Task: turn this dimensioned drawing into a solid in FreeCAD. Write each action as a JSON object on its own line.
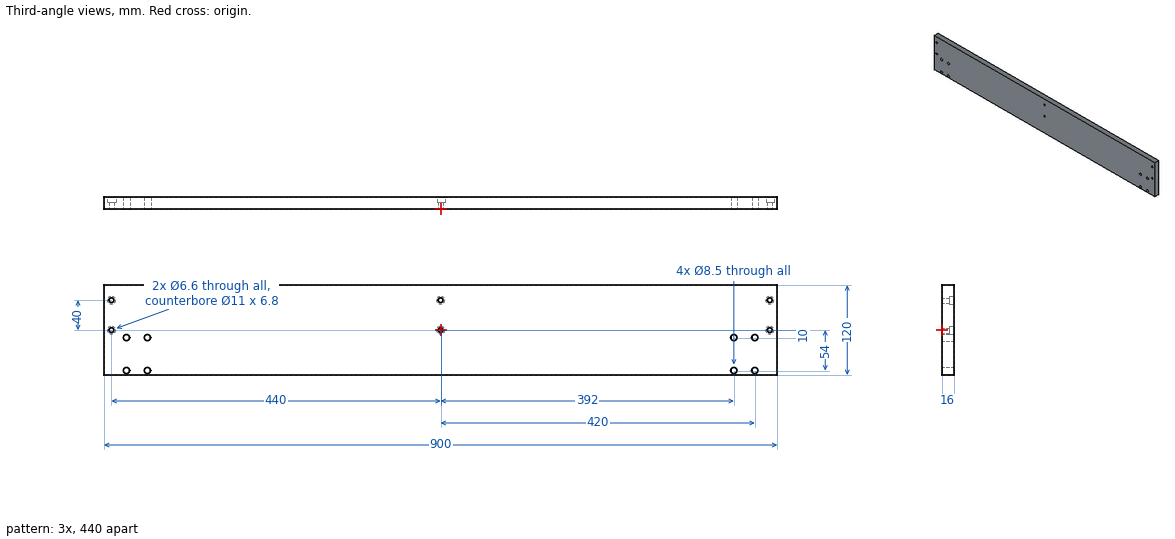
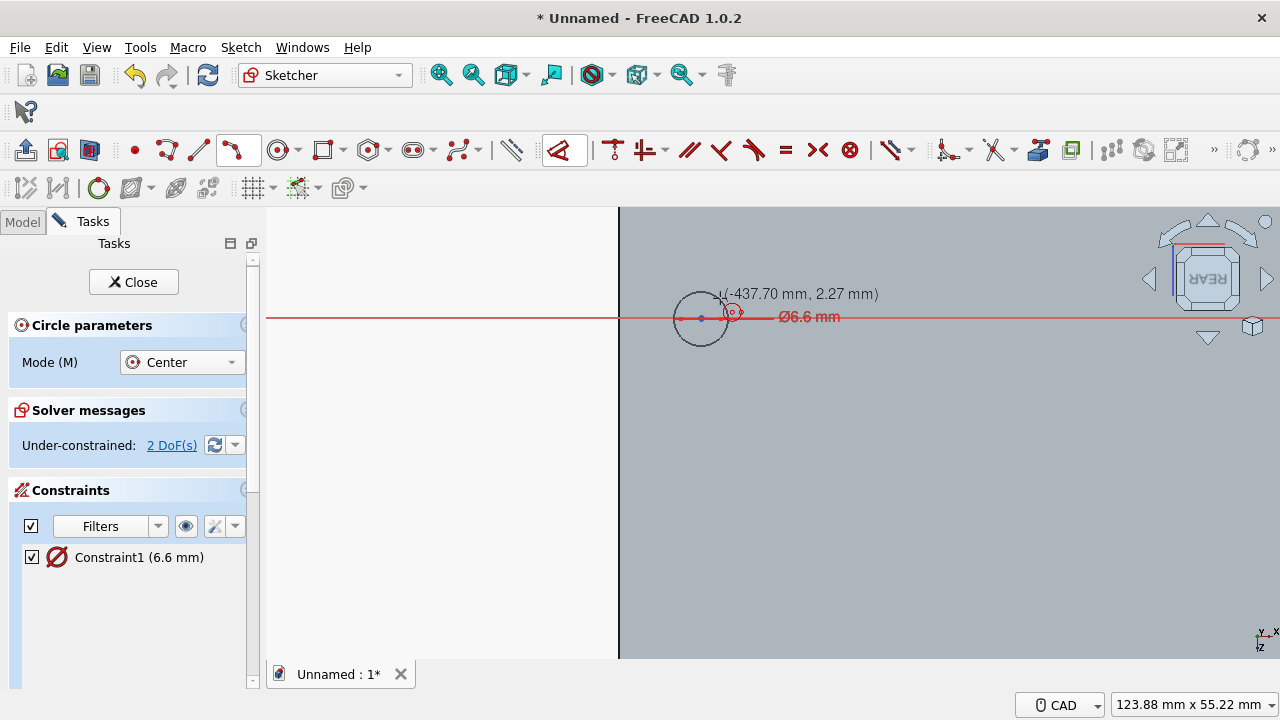
{"action": "scroll", "coordinate": [711, 335], "scroll_direction": "down", "scroll_amount": 2}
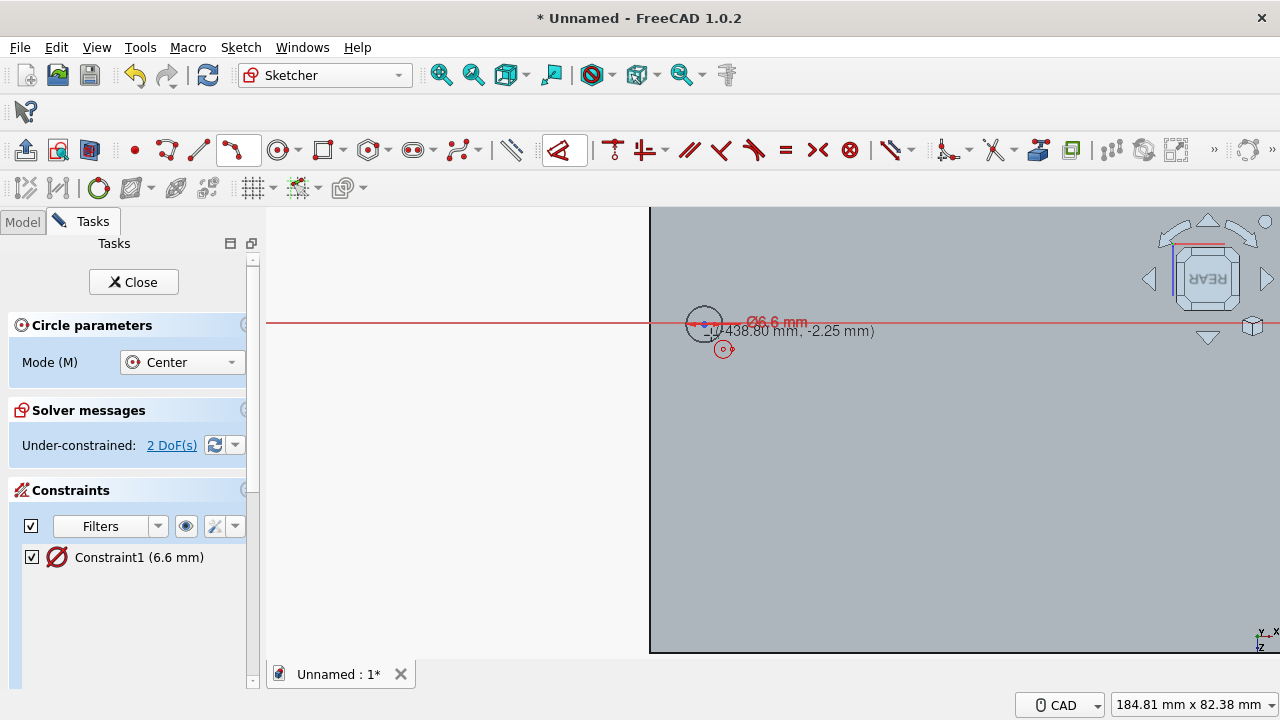
{"action": "scroll", "coordinate": [705, 543], "scroll_direction": "up", "scroll_amount": 2}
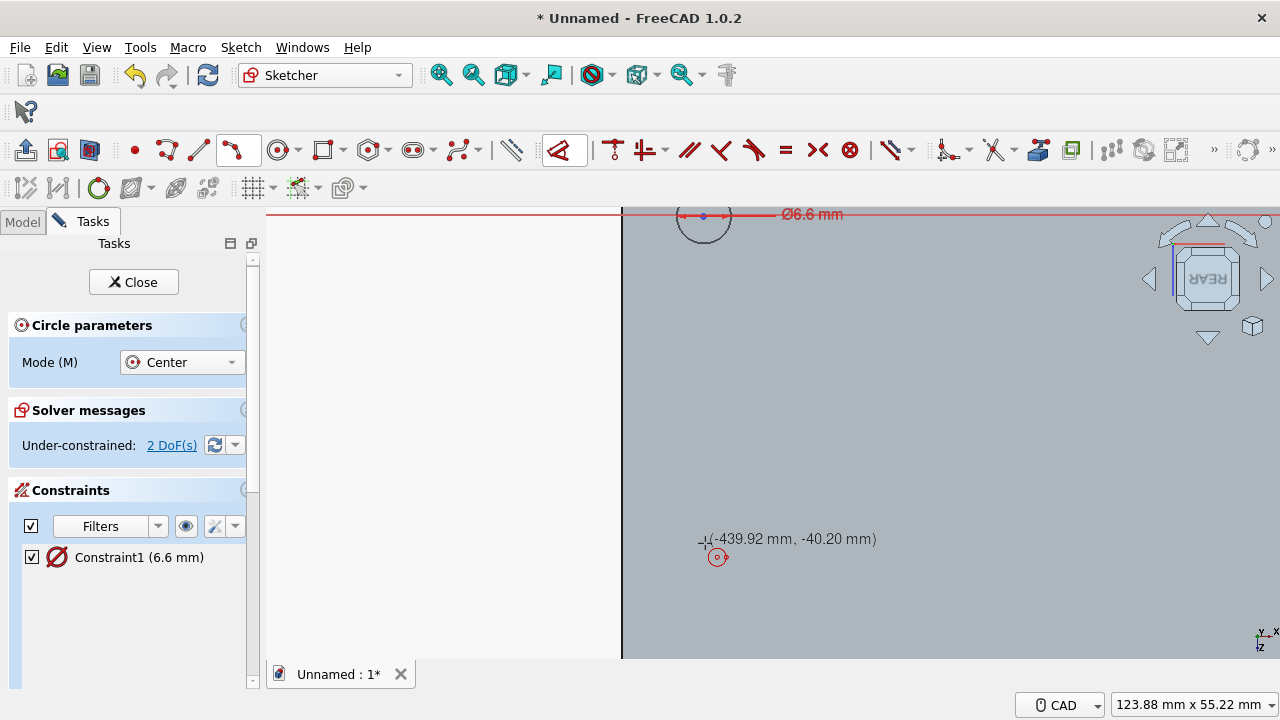
{"action": "left_click", "coordinate": [704, 542]}
{"action": "mouse_move", "coordinate": [723, 523]}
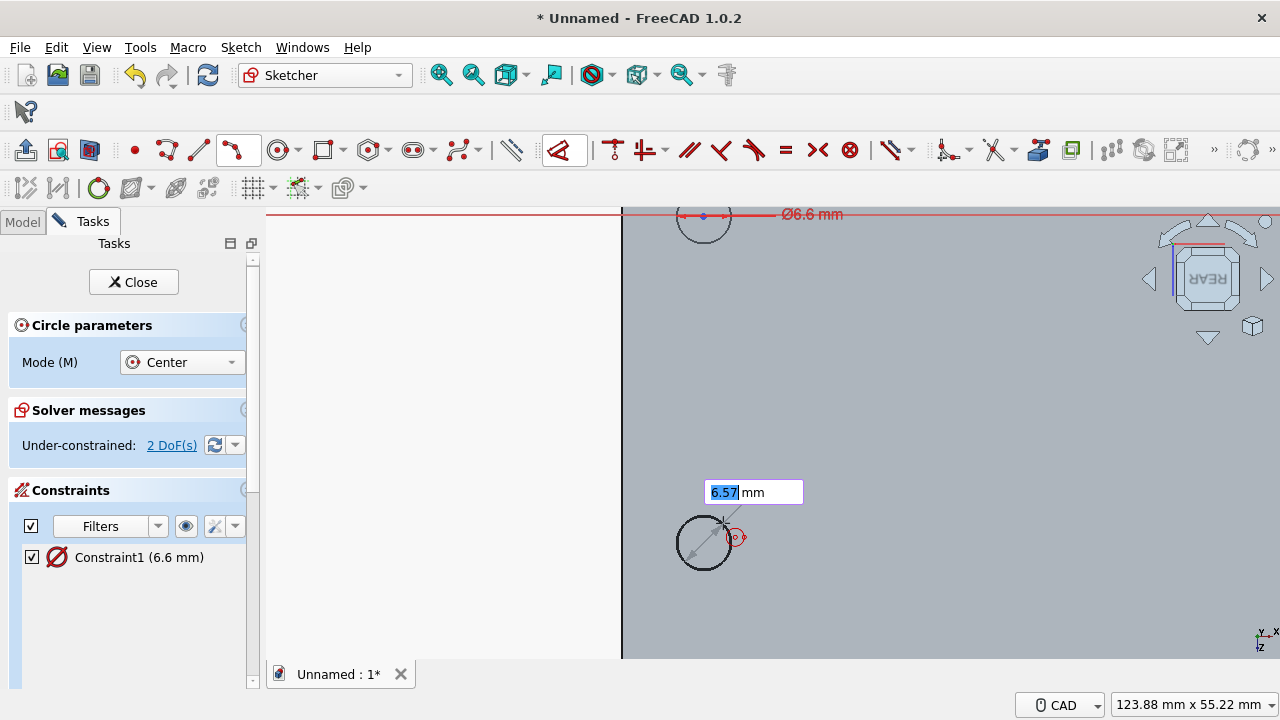
{"action": "type", "text": "6.6"}
{"action": "key", "text": "Return"}
{"action": "key", "text": "Escape"}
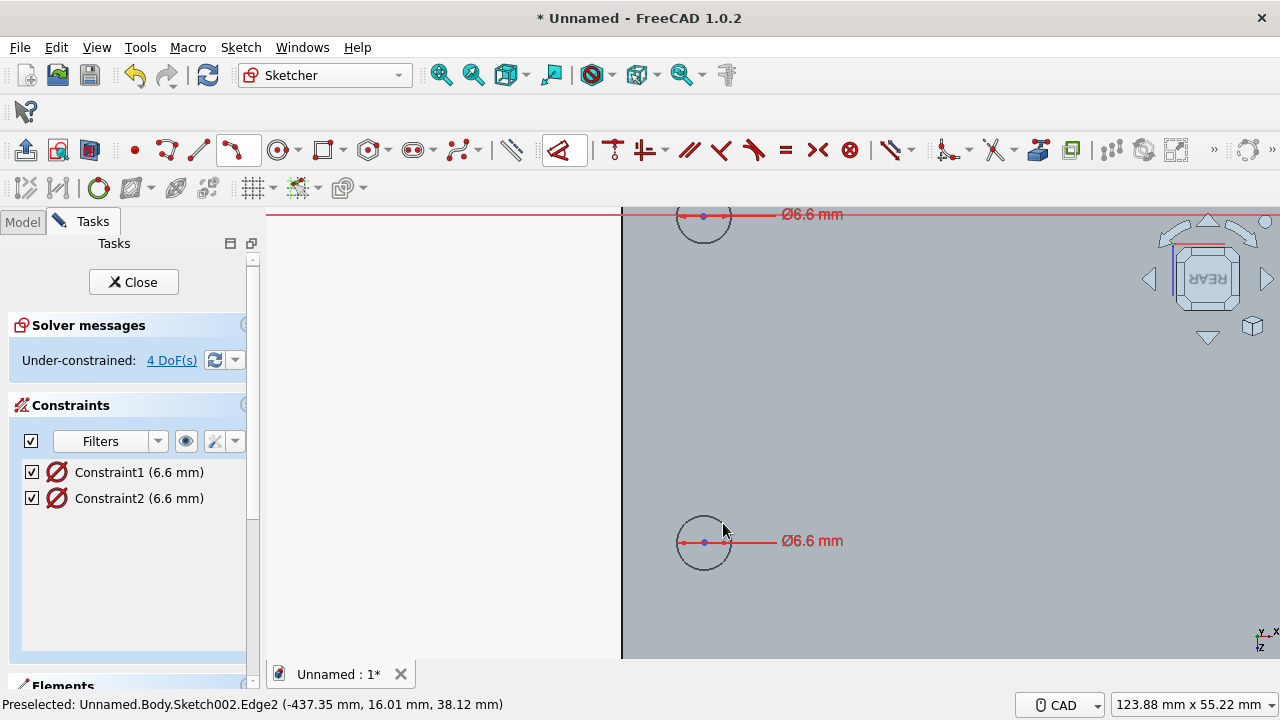
{"action": "scroll", "coordinate": [705, 543], "scroll_direction": "down", "scroll_amount": 2}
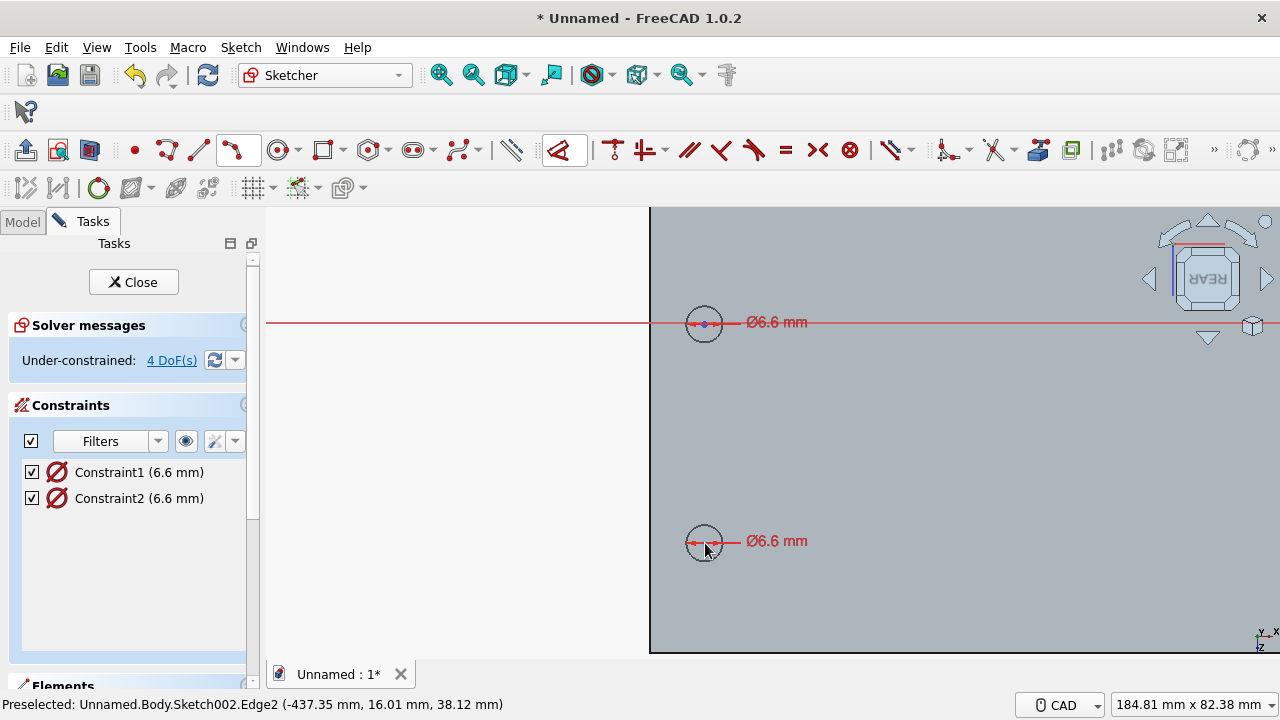
{"action": "left_click", "coordinate": [704, 324]}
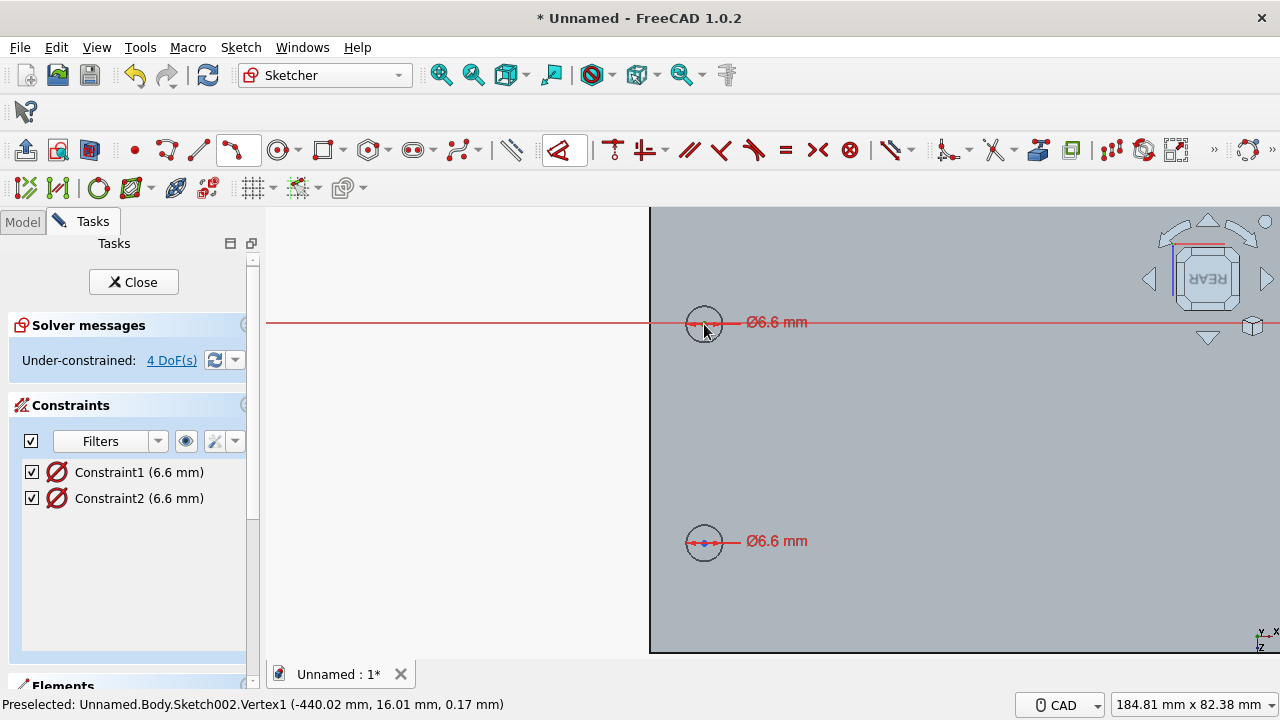
{"action": "left_click", "coordinate": [353, 323]}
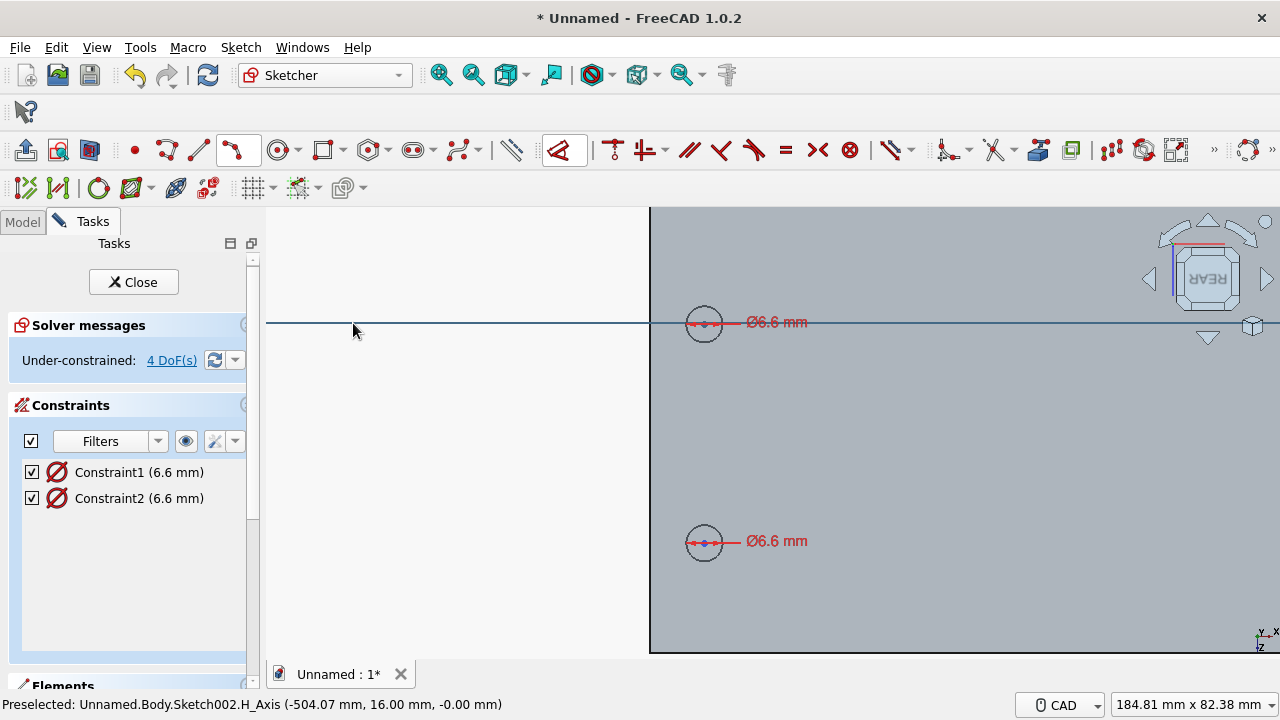
{"action": "key", "text": "c"}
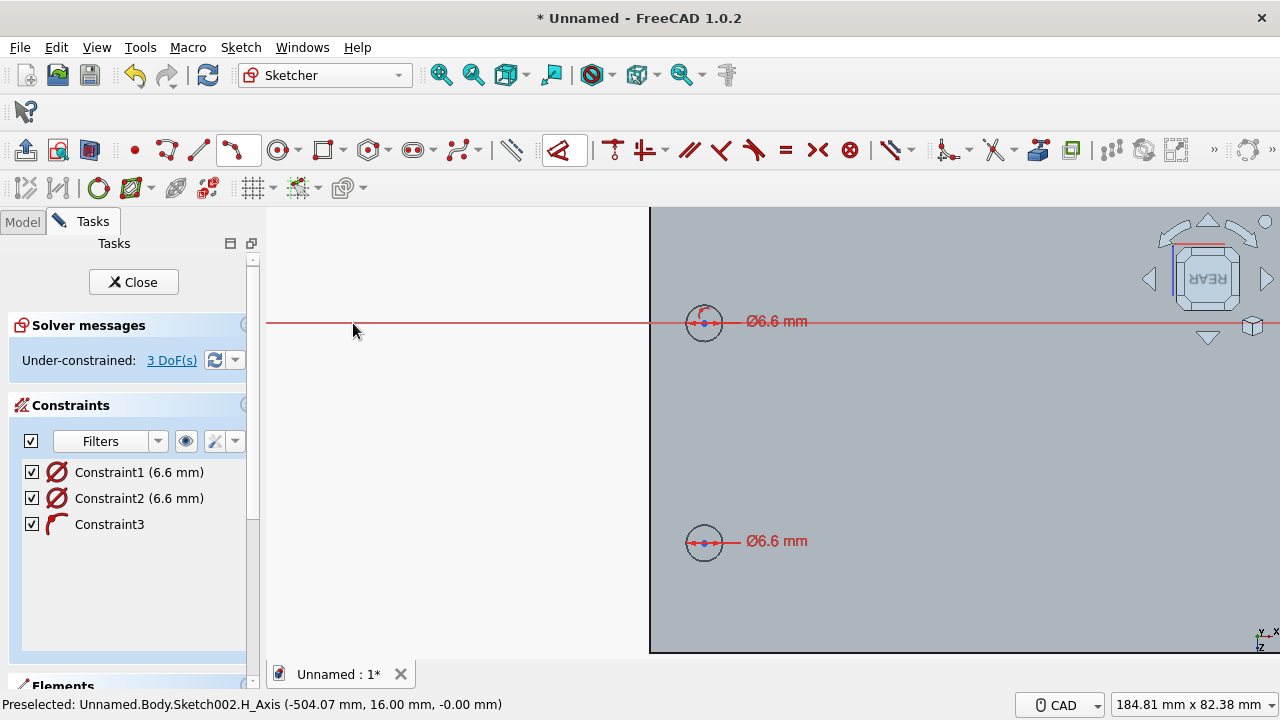
{"action": "left_click", "coordinate": [704, 543]}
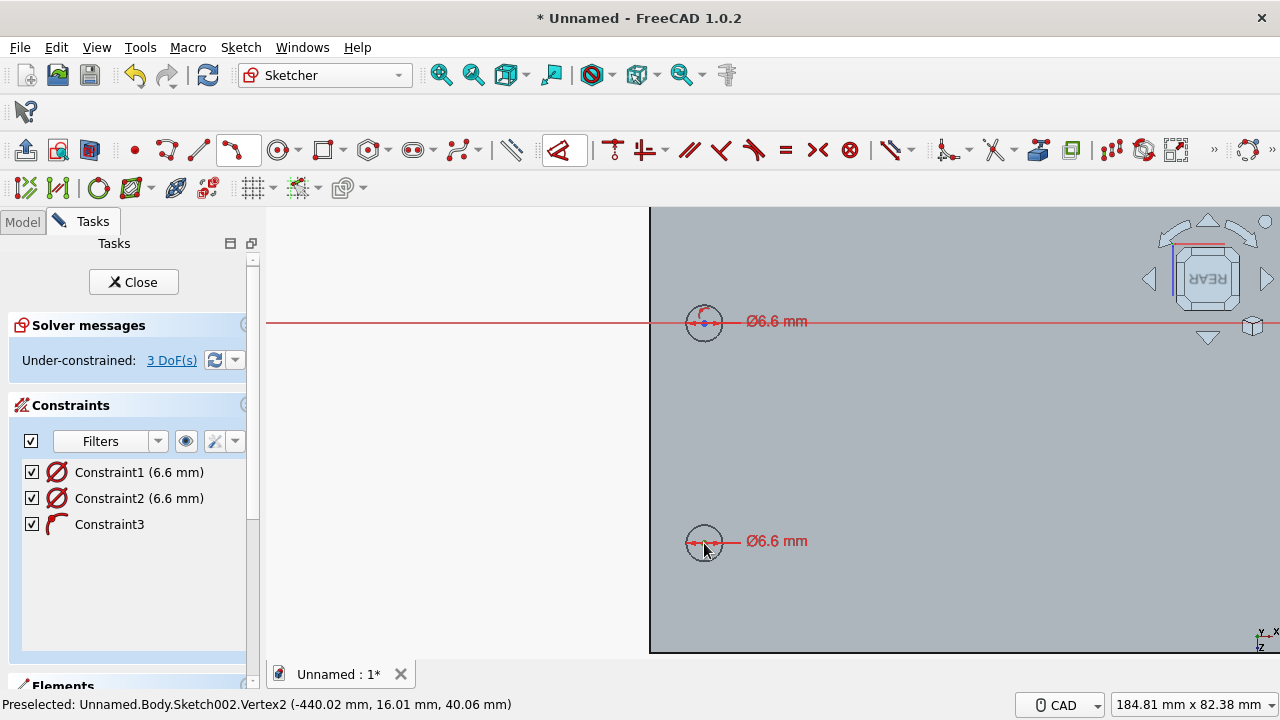
{"action": "left_click", "coordinate": [582, 150]}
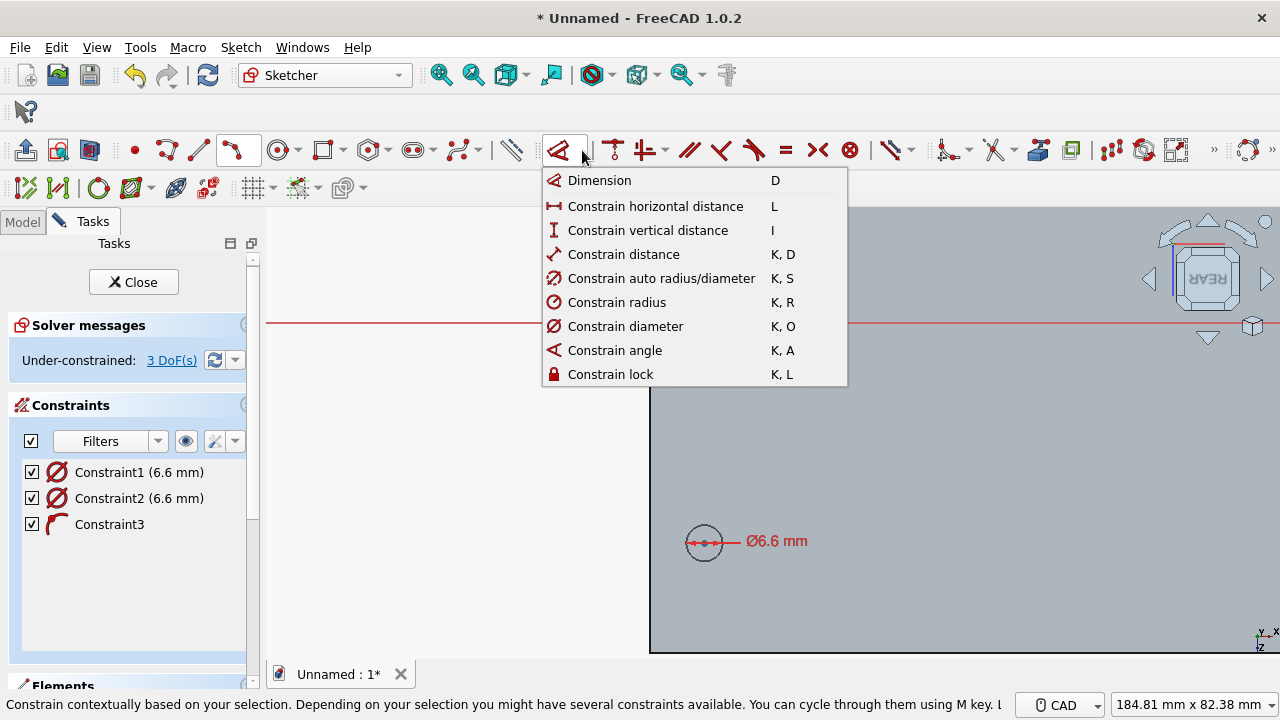
{"action": "left_click", "coordinate": [695, 230]}